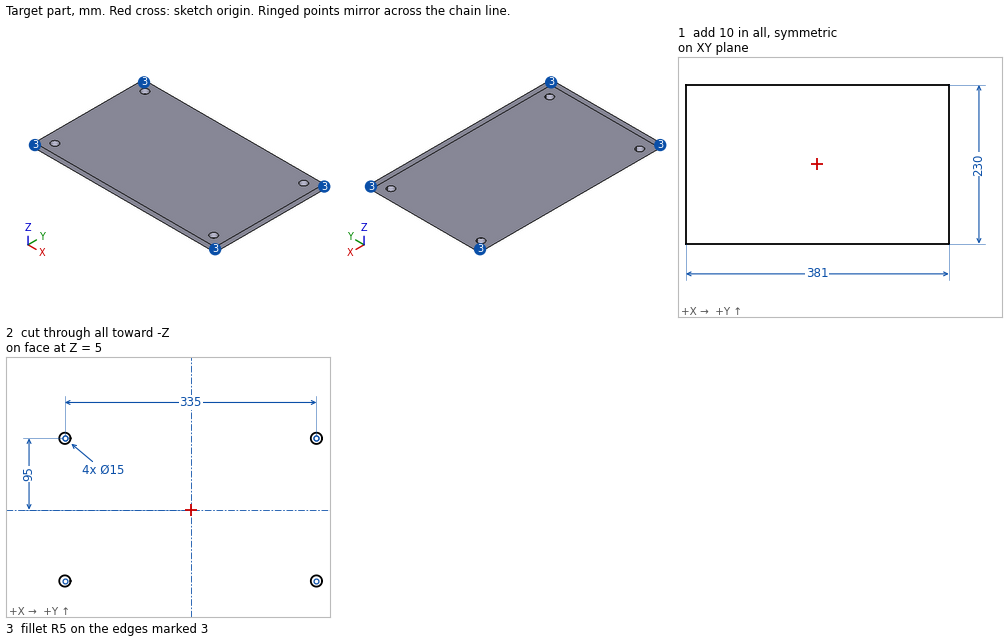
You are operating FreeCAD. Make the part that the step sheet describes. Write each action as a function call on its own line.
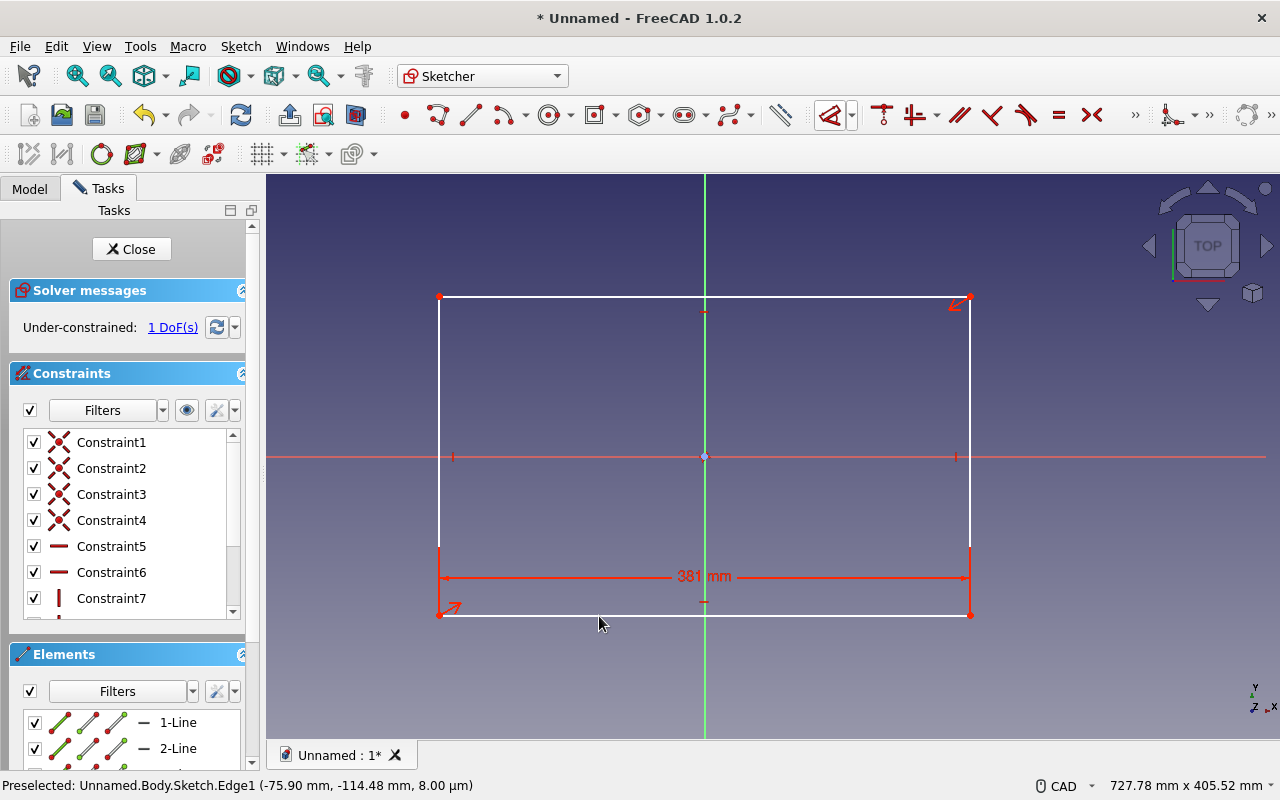
click(970, 520)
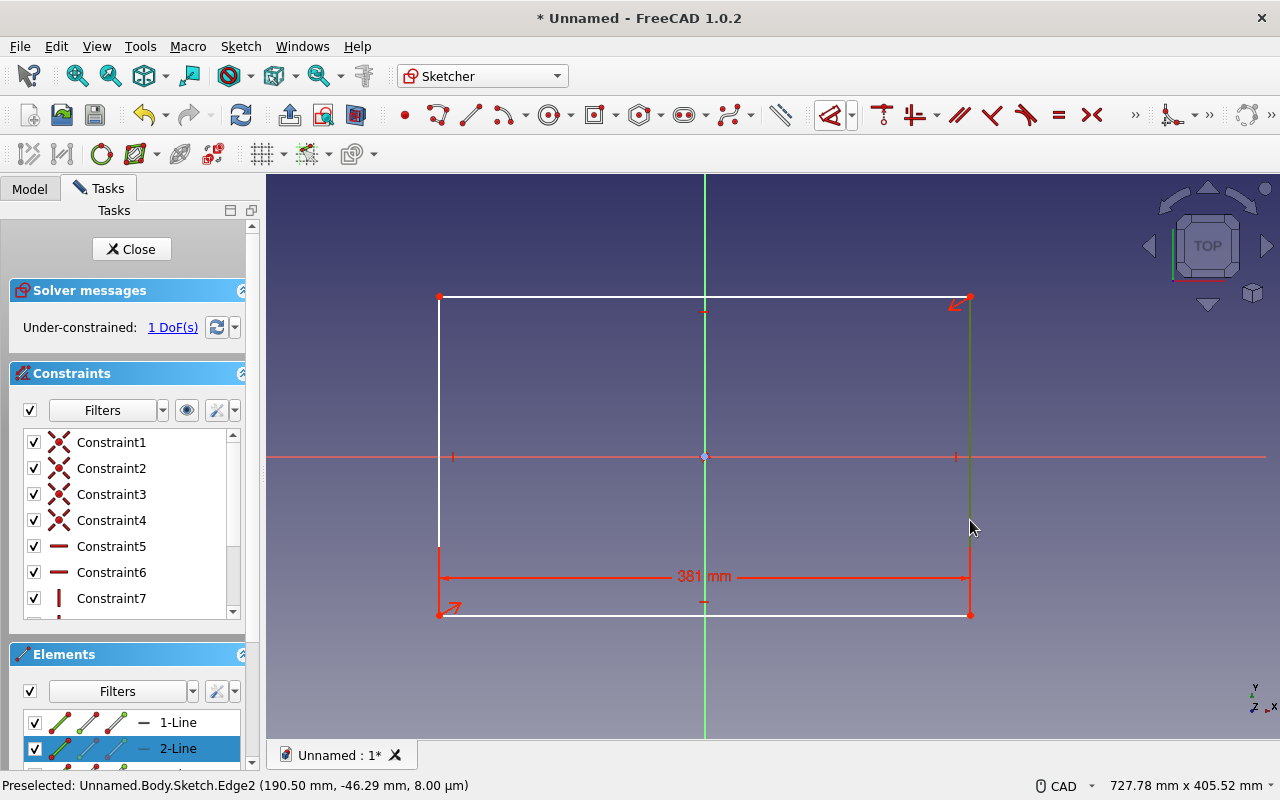
click(852, 116)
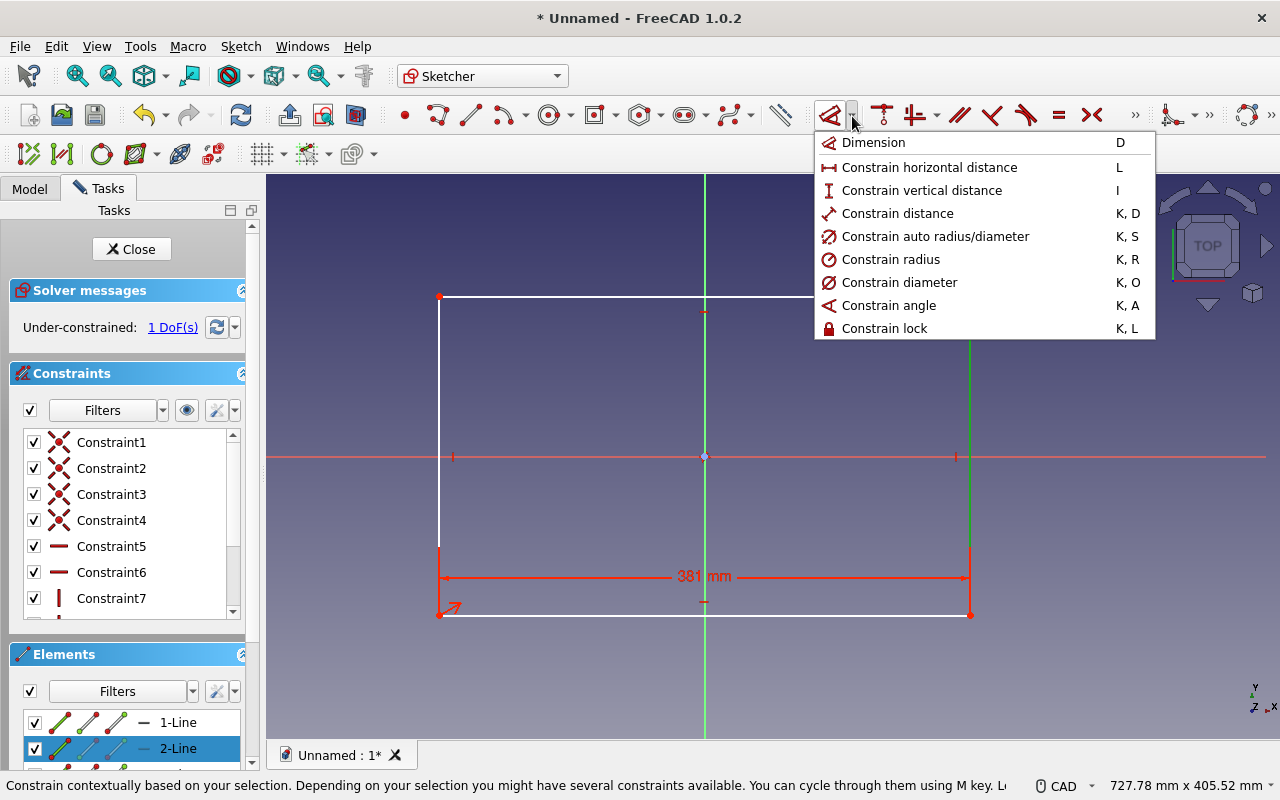
click(985, 190)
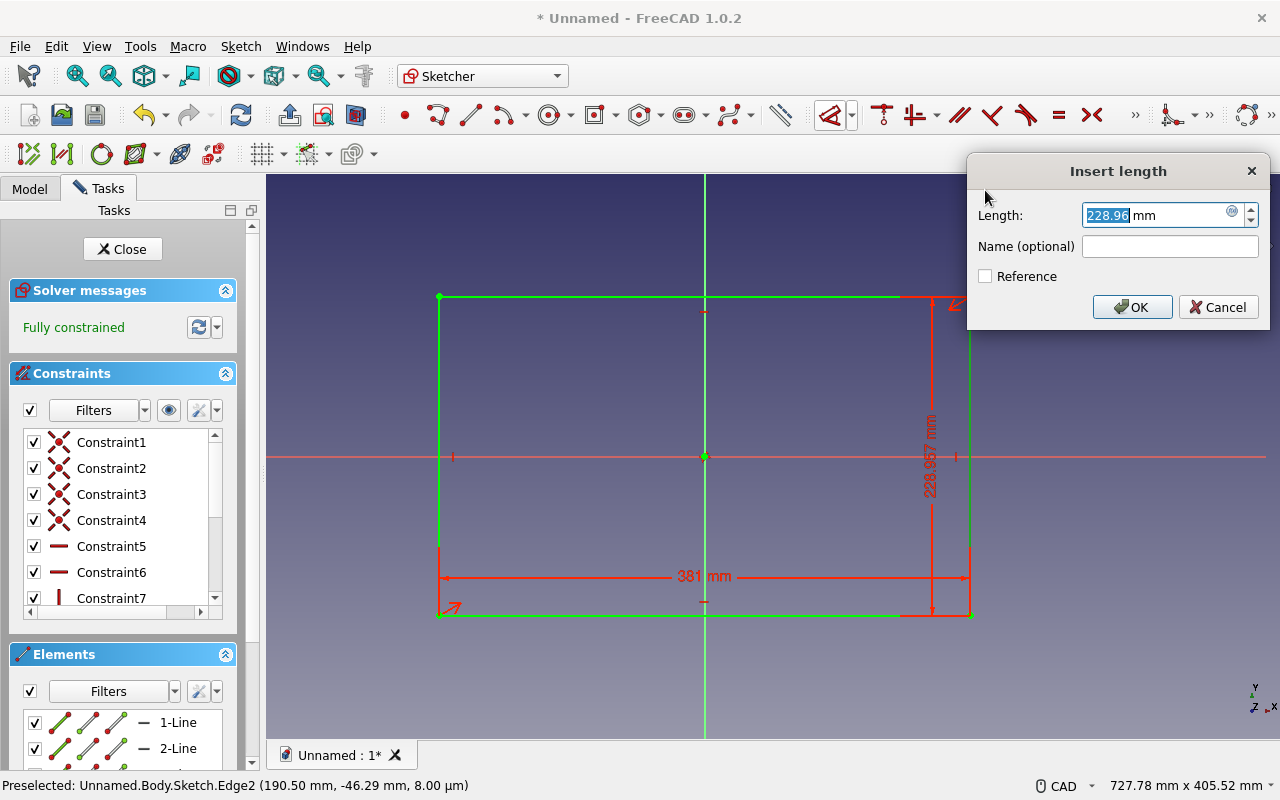
text(230)
key(Return)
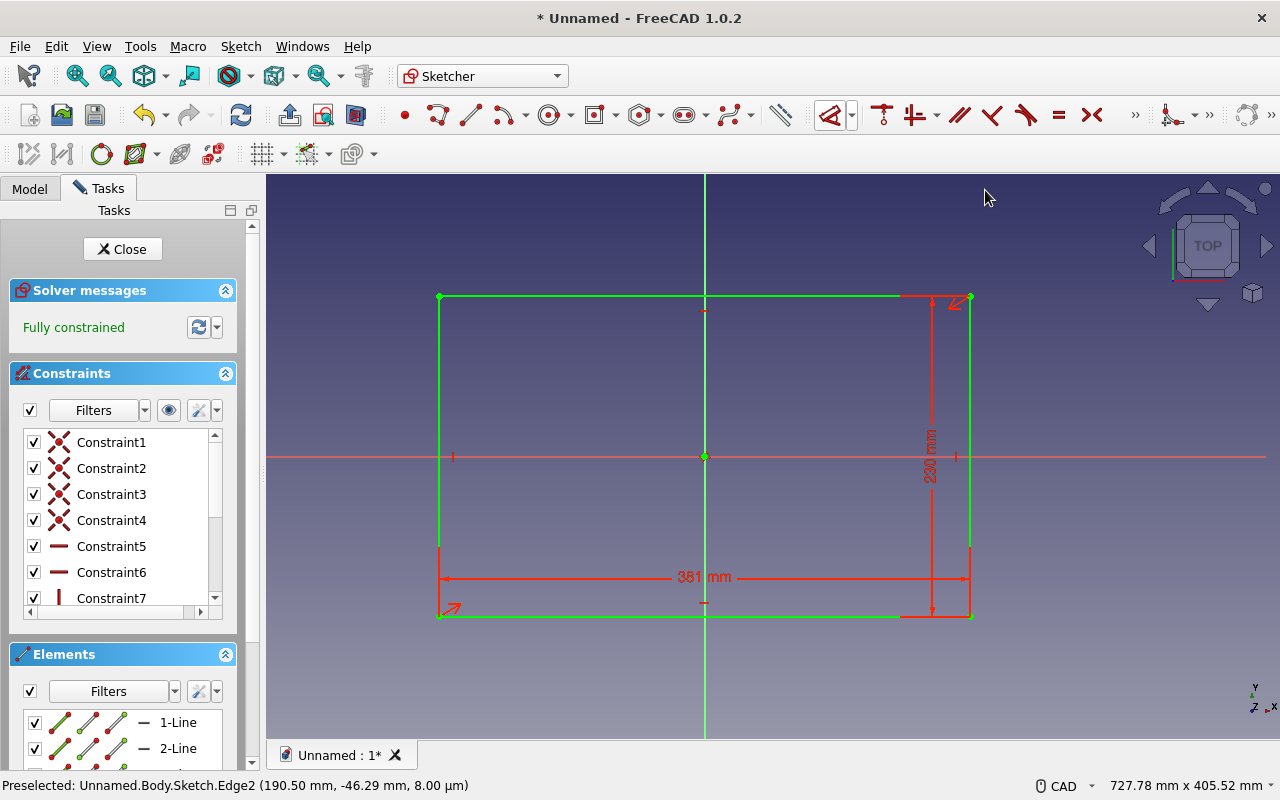
click(123, 249)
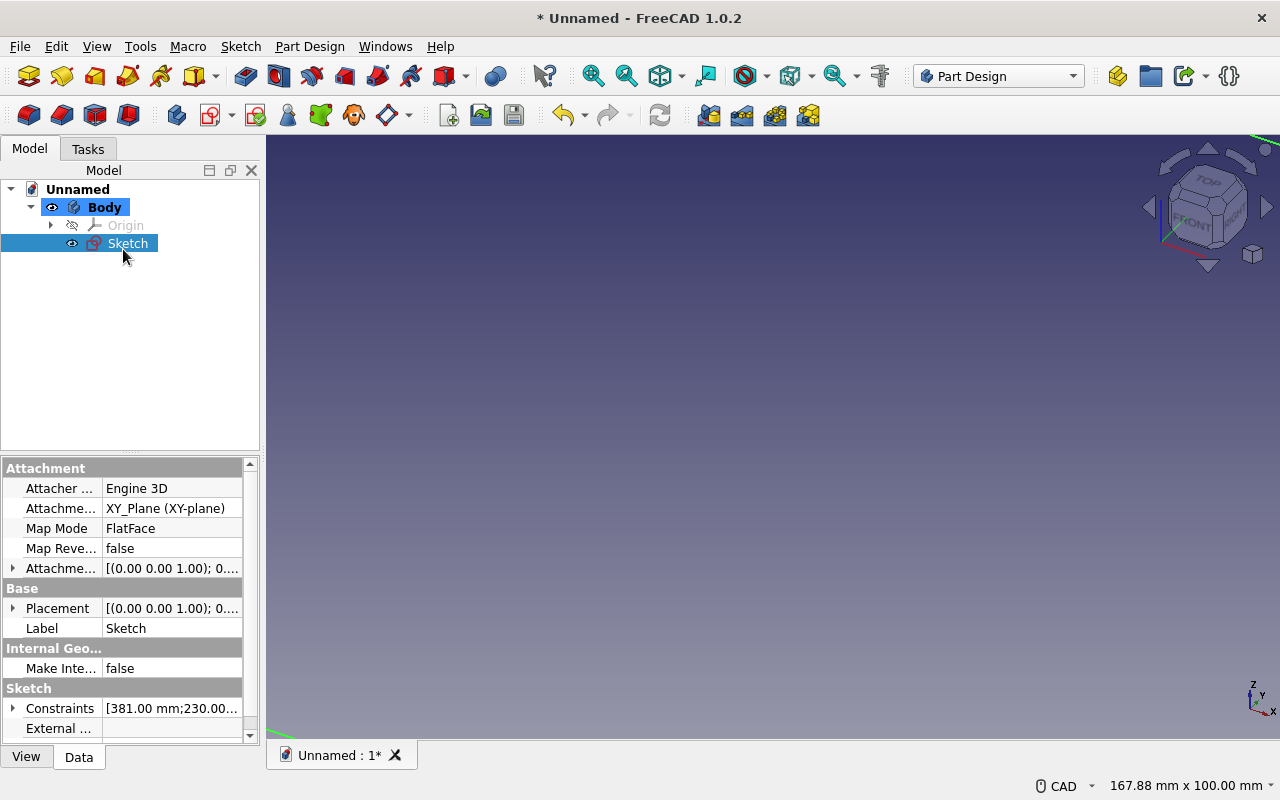
click(29, 76)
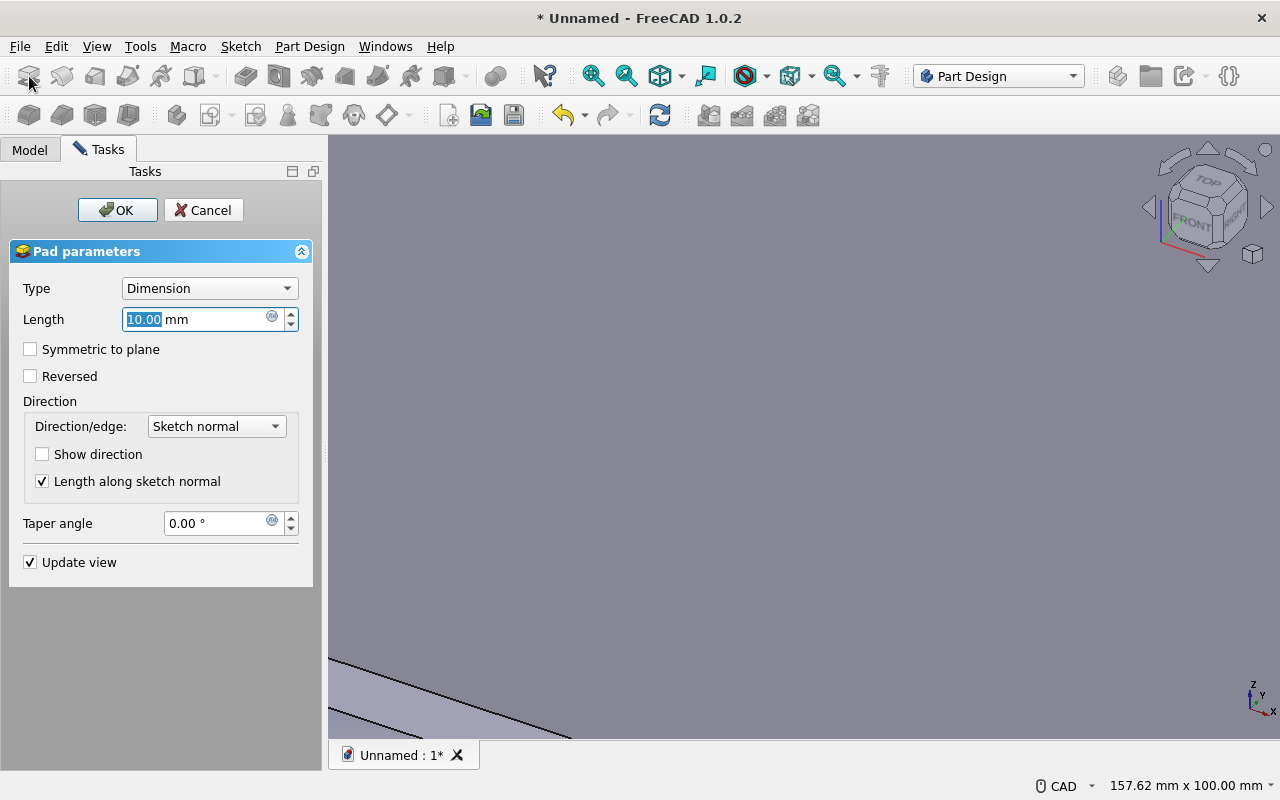
text(10)
key(Tab)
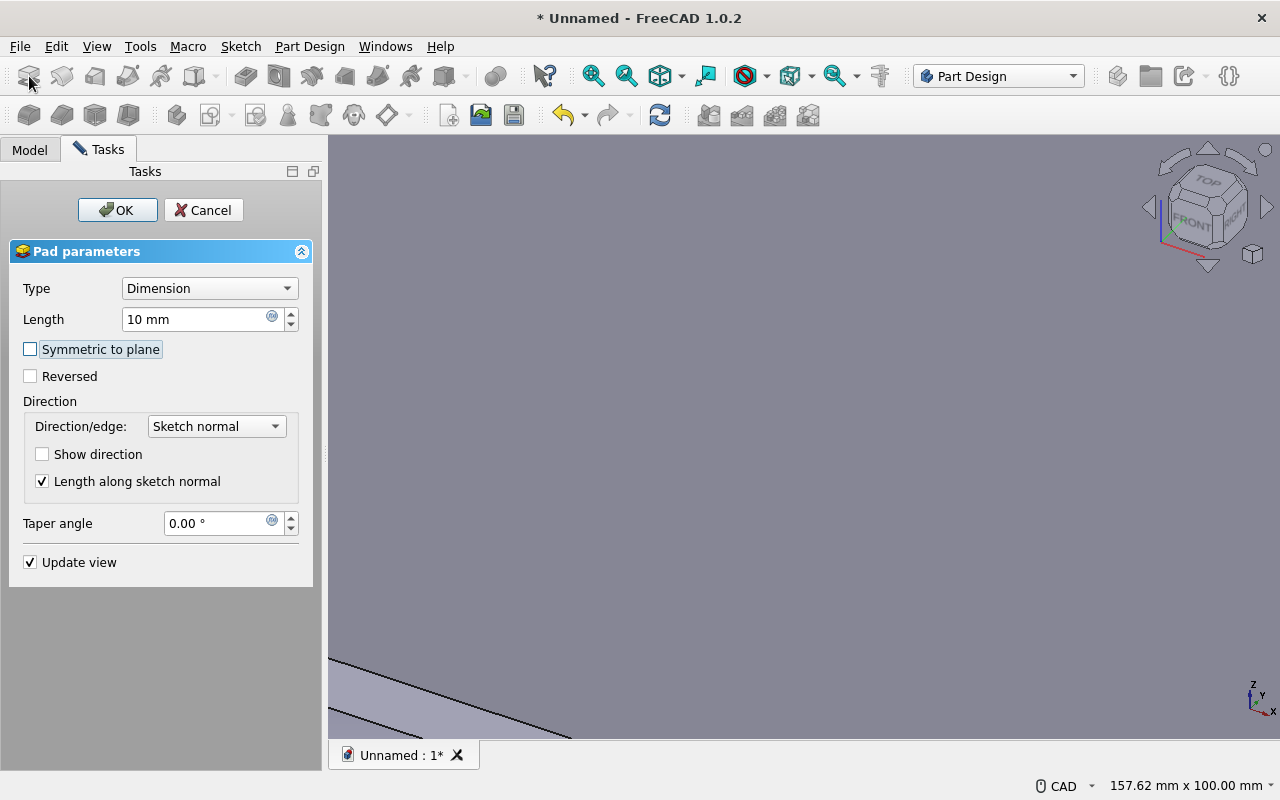
click(31, 349)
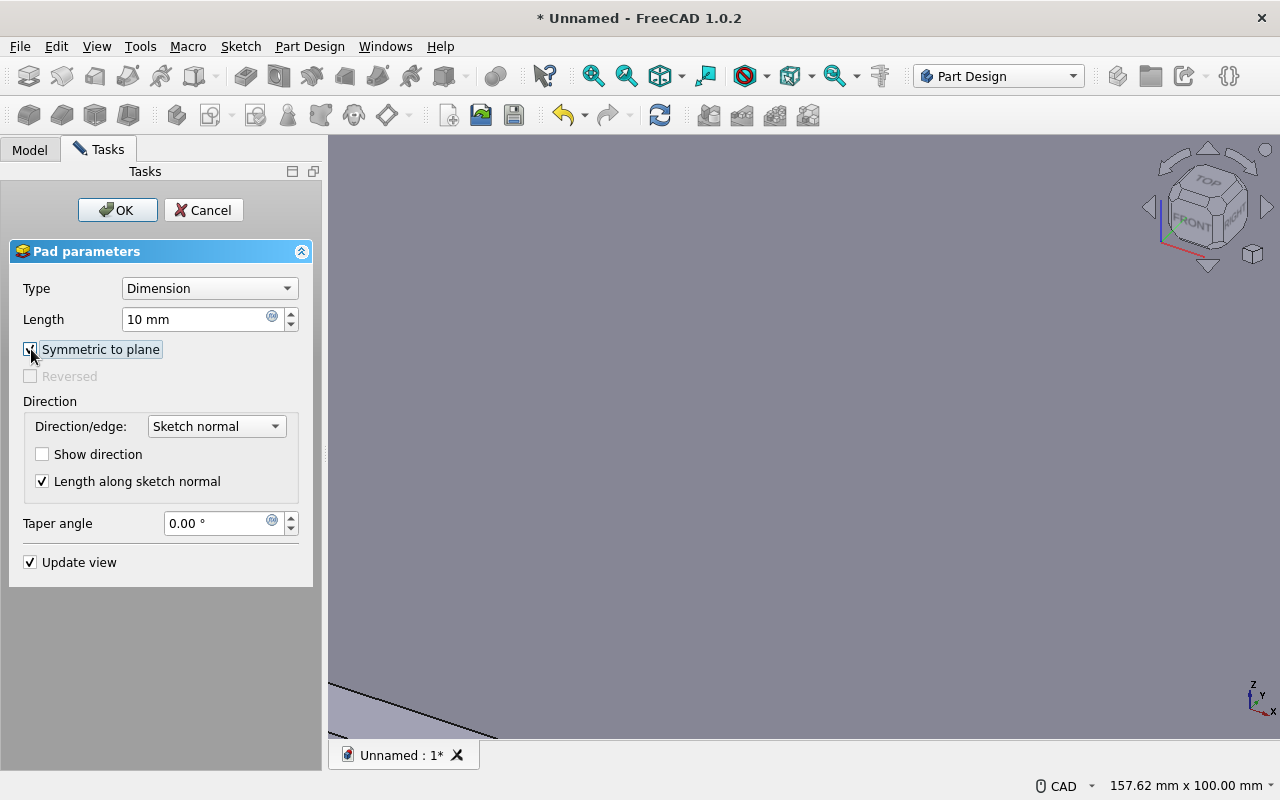
click(118, 210)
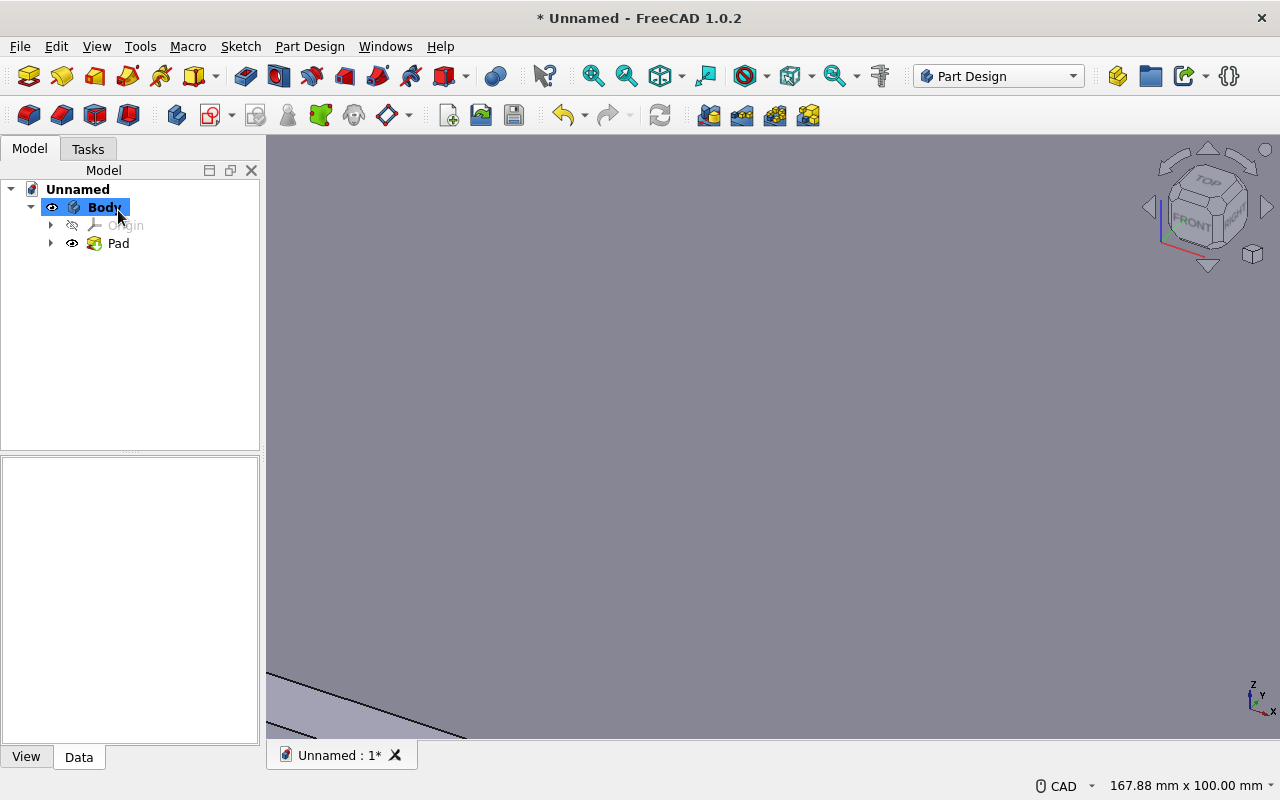
key(v)
key(f)